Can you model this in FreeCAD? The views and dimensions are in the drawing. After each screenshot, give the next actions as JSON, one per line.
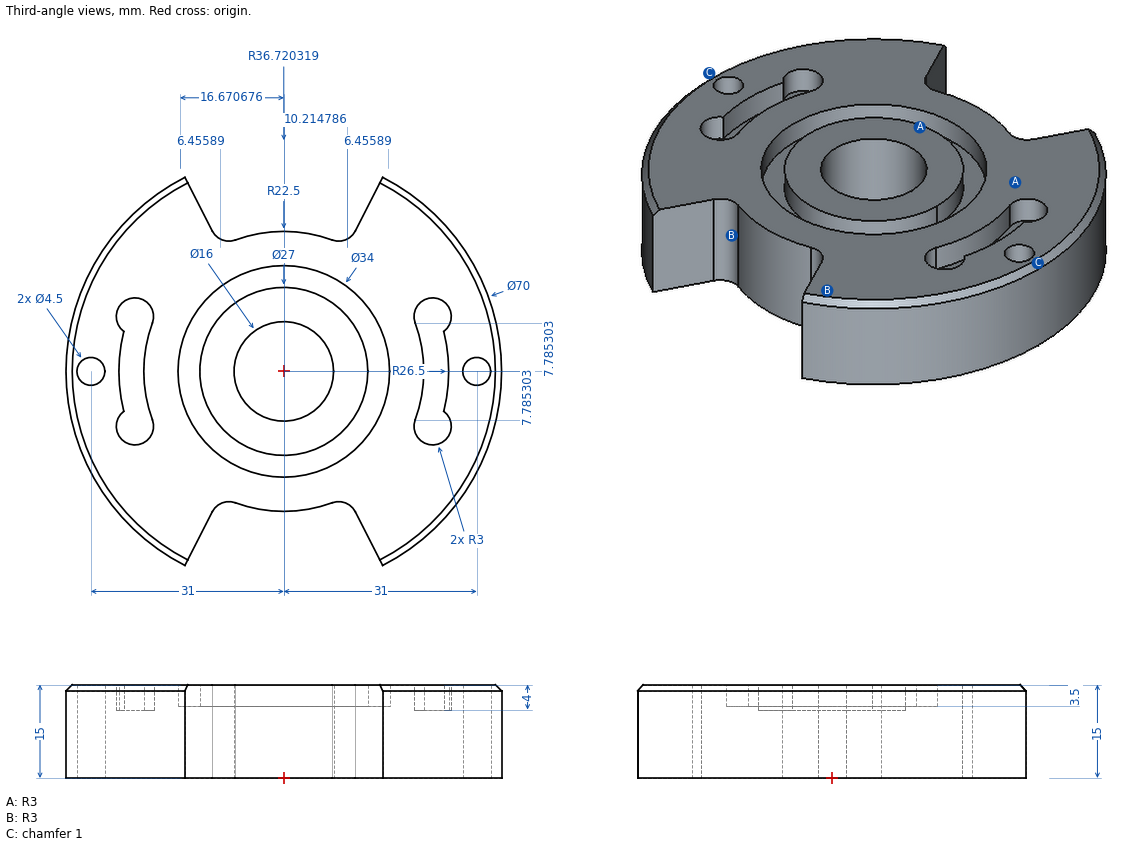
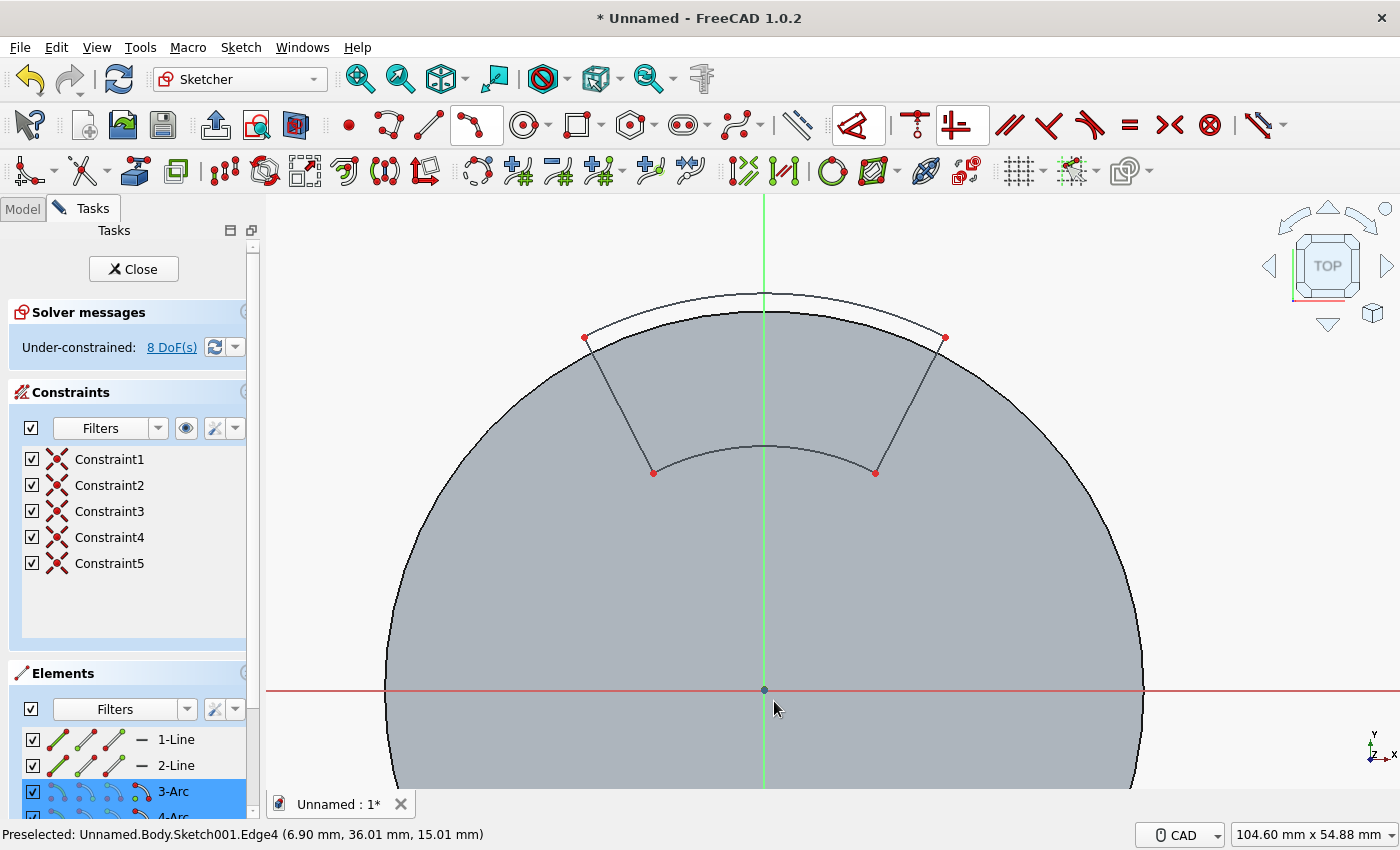
{"action": "left_click", "coordinate": [916, 126]}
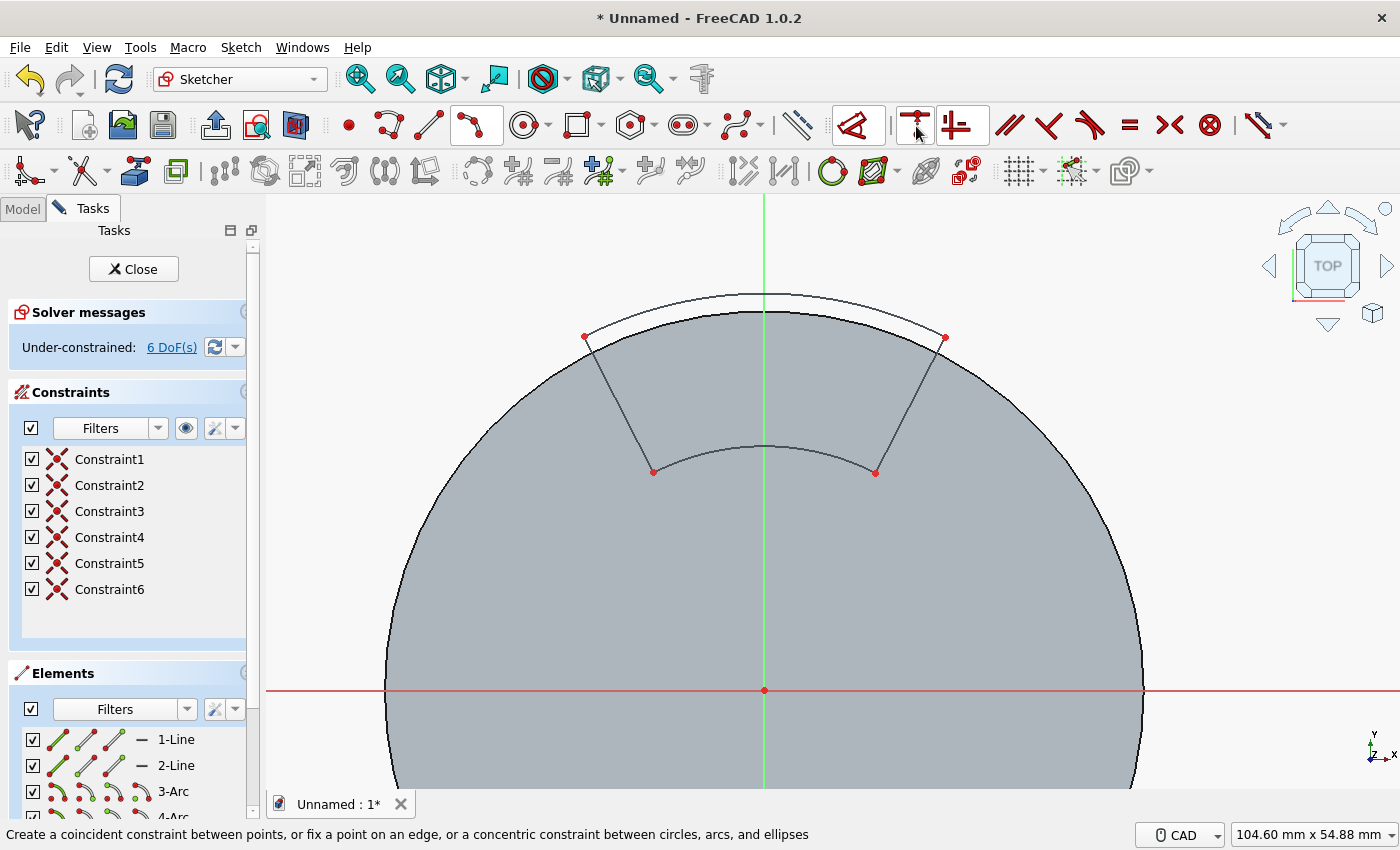
{"action": "left_click", "coordinate": [852, 126]}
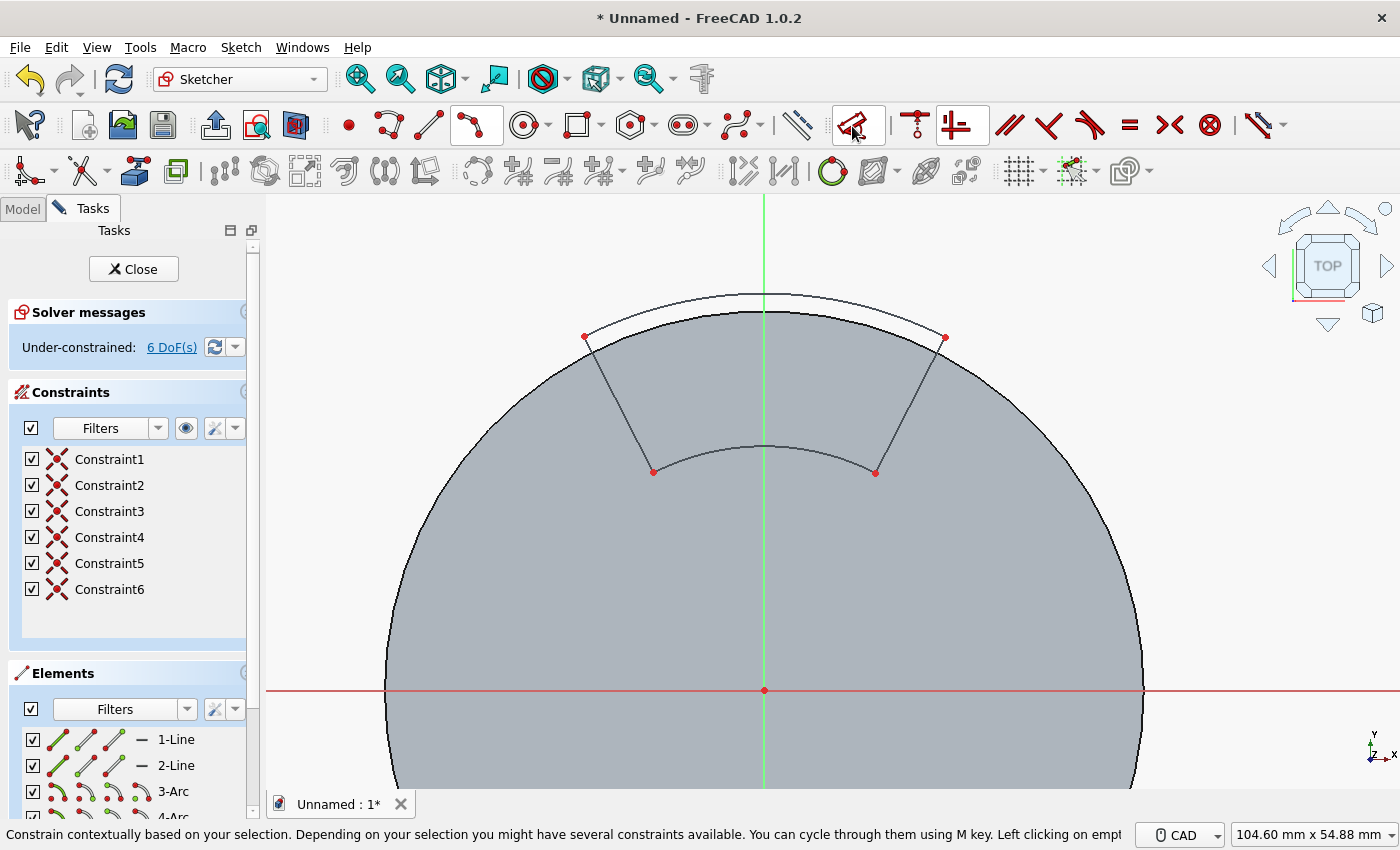
{"action": "left_click", "coordinate": [810, 451]}
{"action": "left_click", "coordinate": [816, 420]}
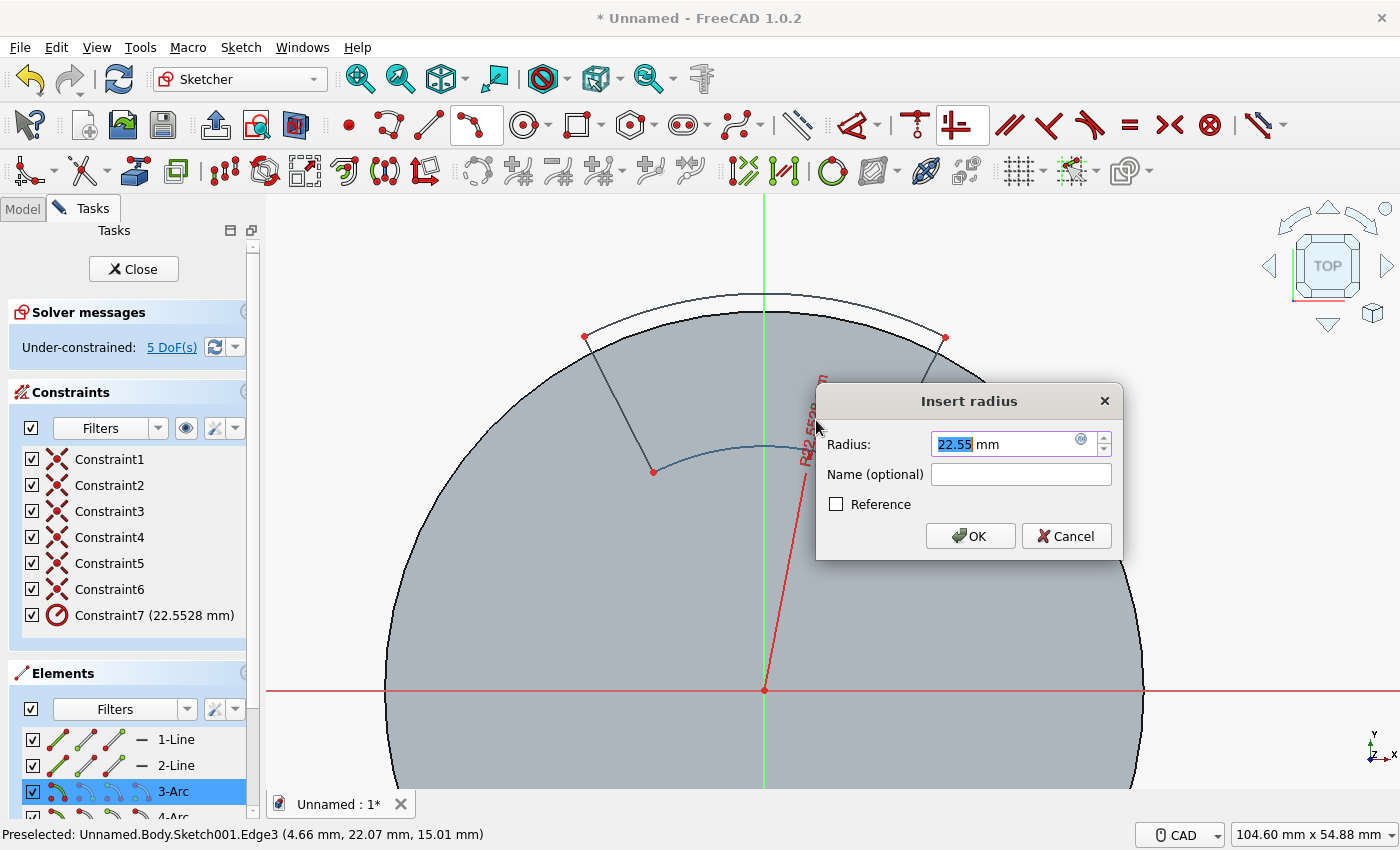
{"action": "type", "text": "22.5"}
{"action": "key", "text": "Return"}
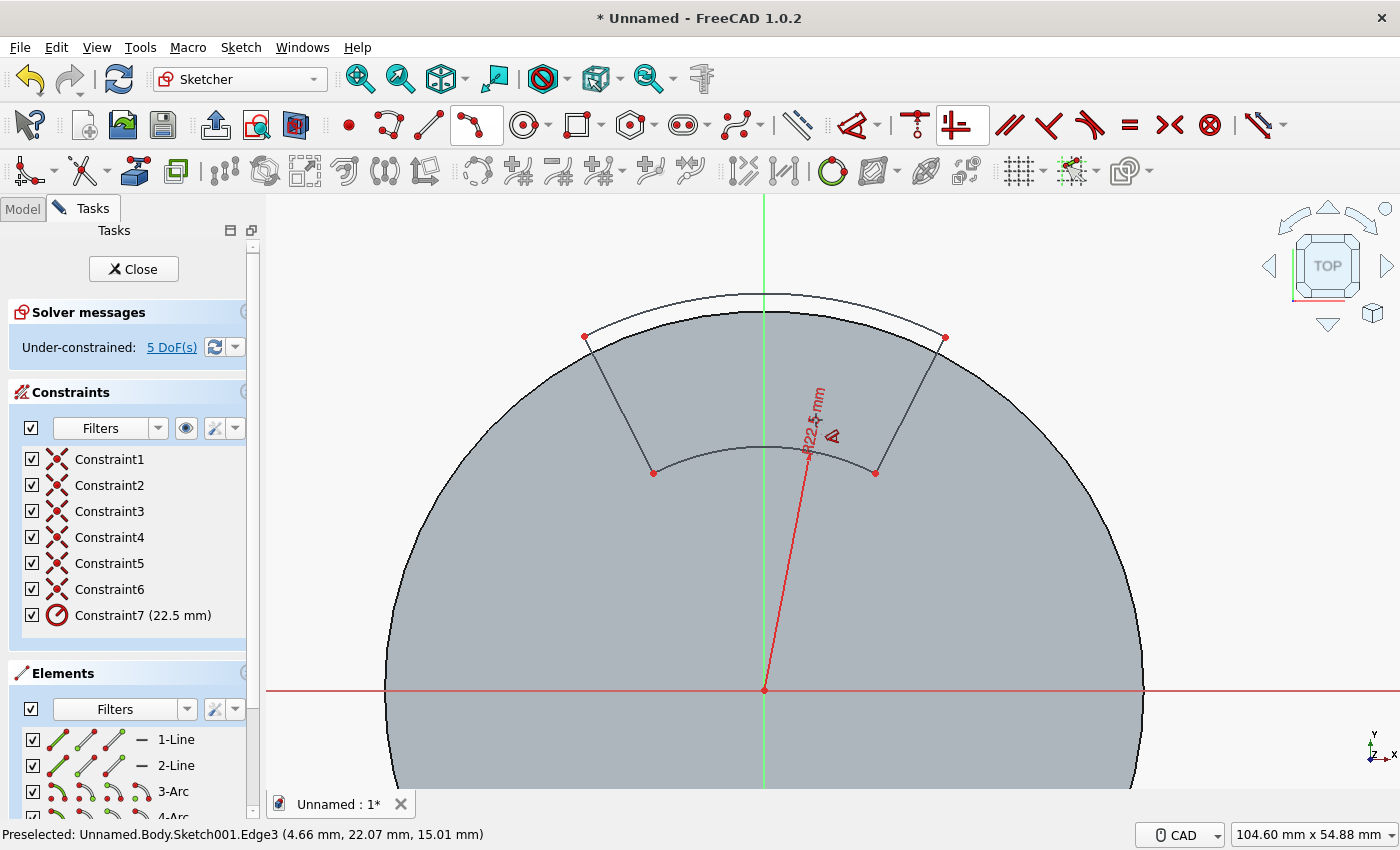
{"action": "left_click", "coordinate": [839, 301]}
{"action": "left_click", "coordinate": [845, 270]}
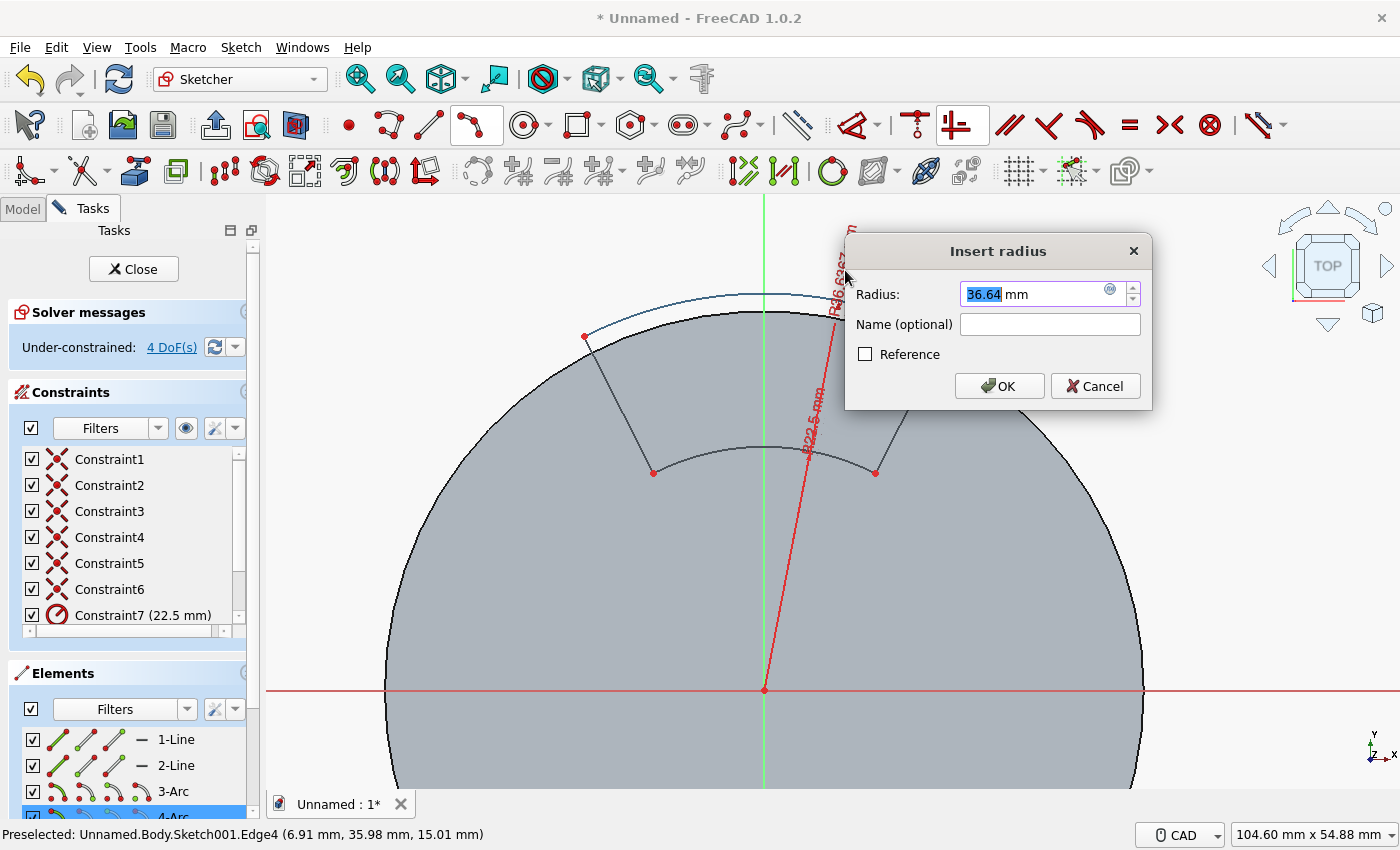
{"action": "type", "text": "36.720319"}
{"action": "key", "text": "Return"}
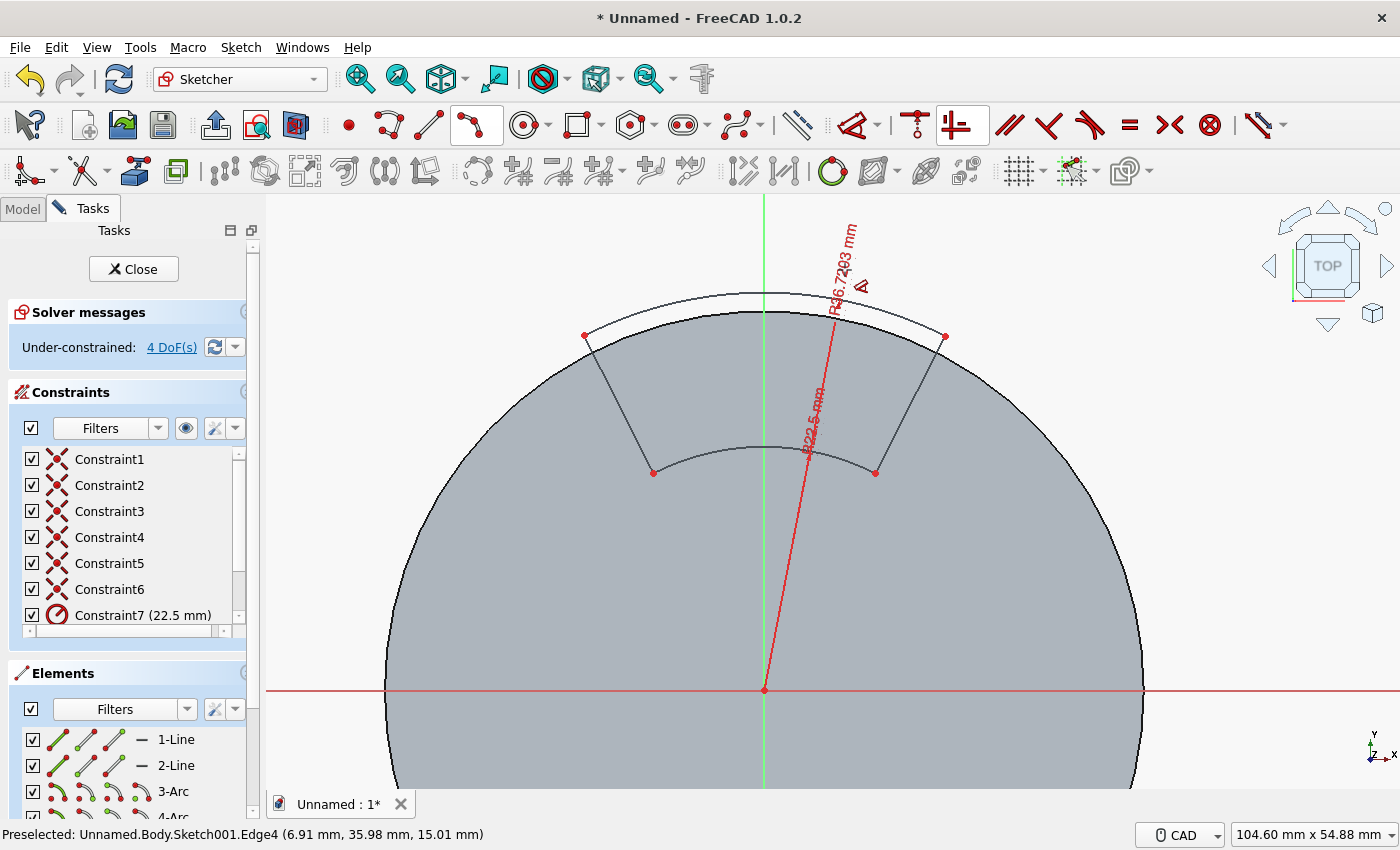
{"action": "left_click", "coordinate": [605, 377]}
{"action": "left_click", "coordinate": [619, 302]}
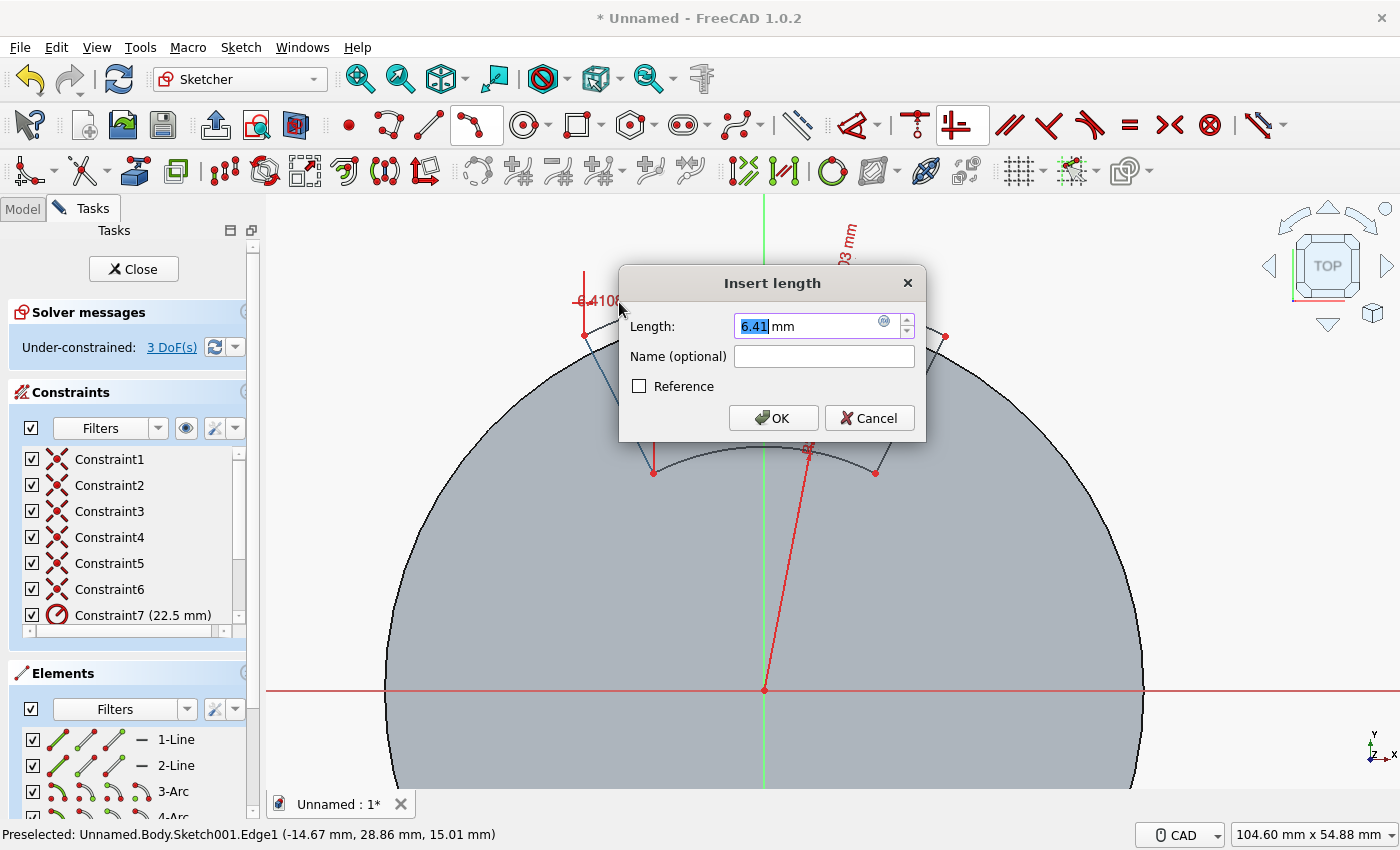
{"action": "type", "text": "6.45589"}
{"action": "key", "text": "Return"}